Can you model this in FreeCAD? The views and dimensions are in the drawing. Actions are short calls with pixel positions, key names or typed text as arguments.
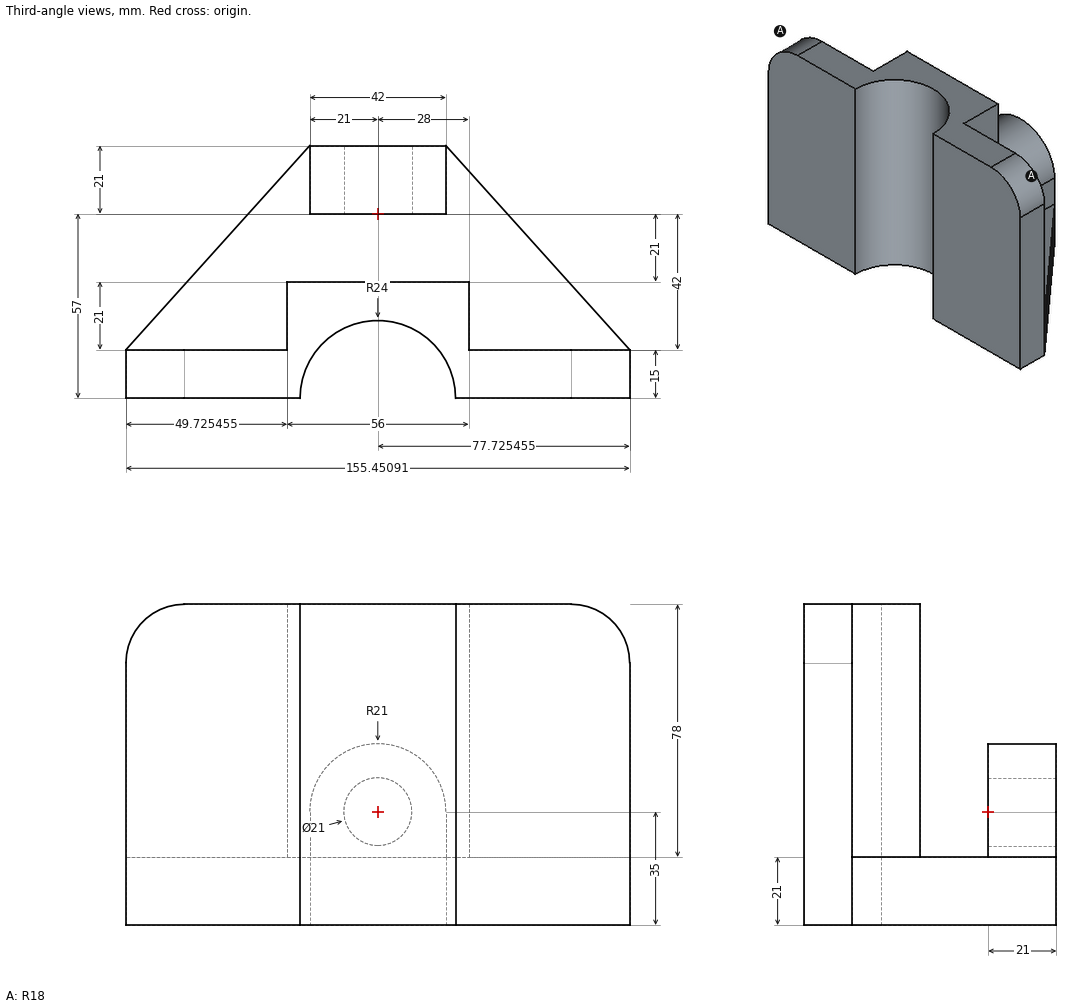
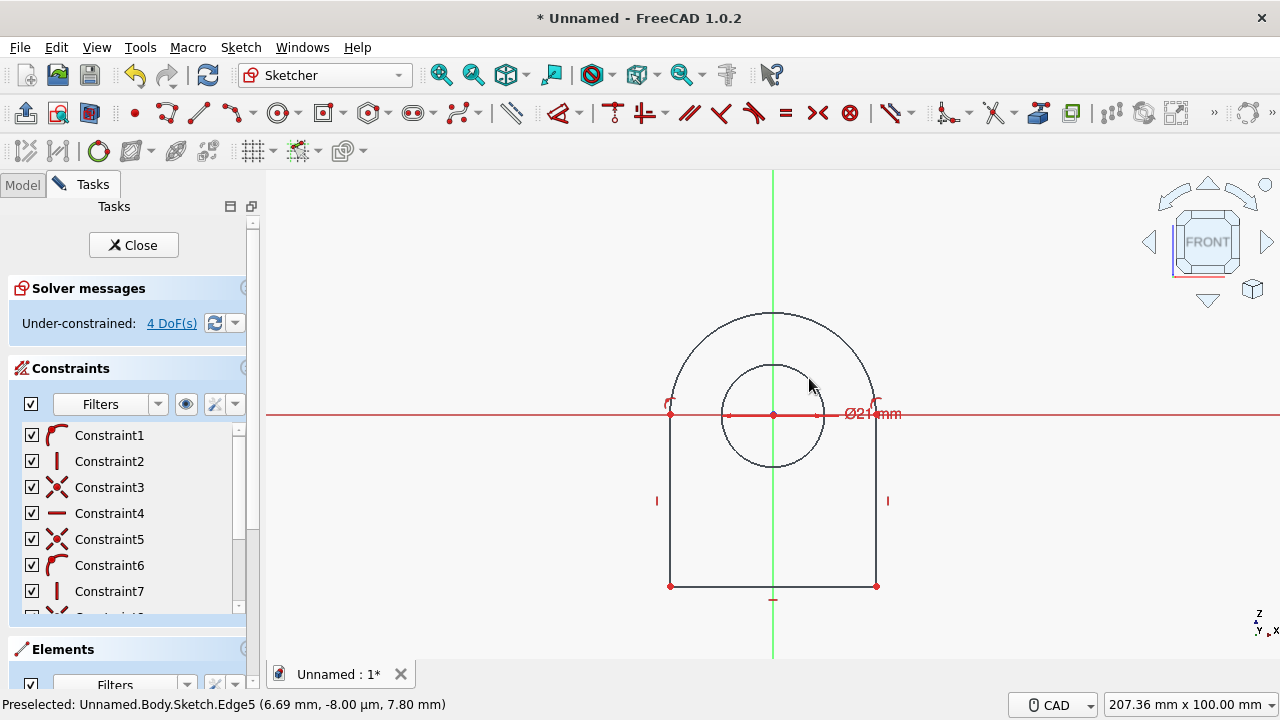
click(876, 466)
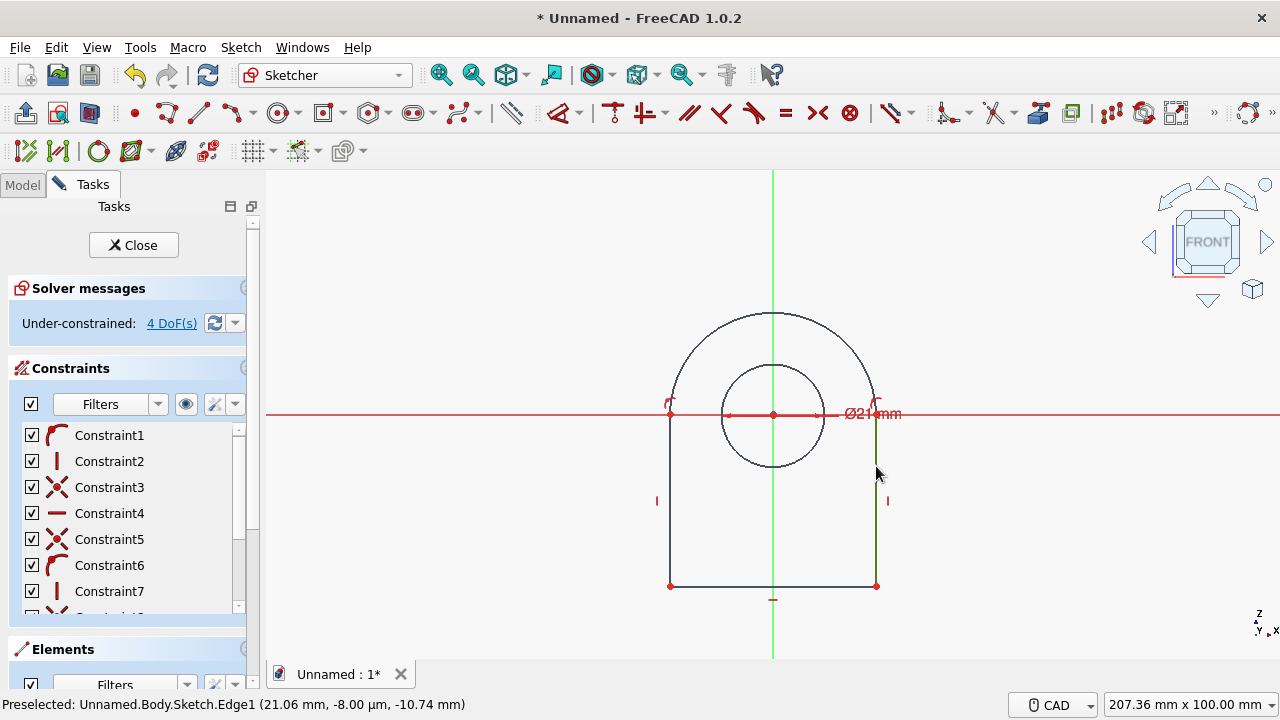
click(833, 332)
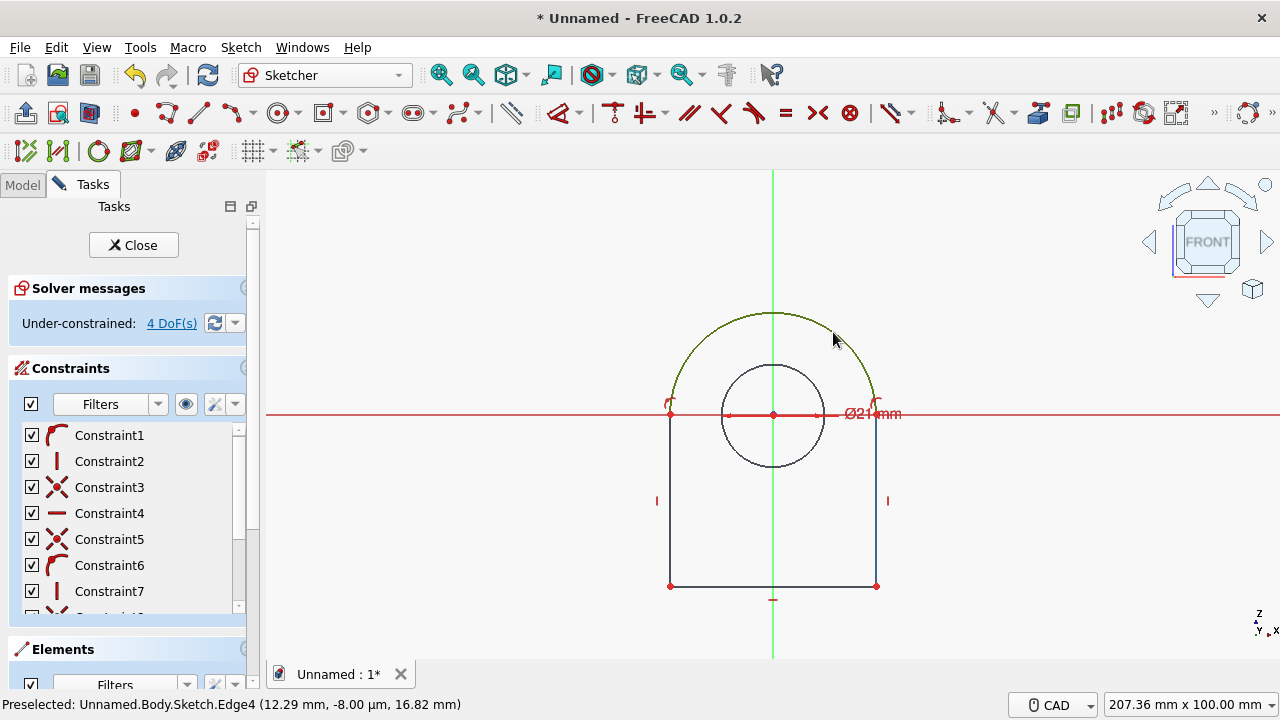
click(754, 114)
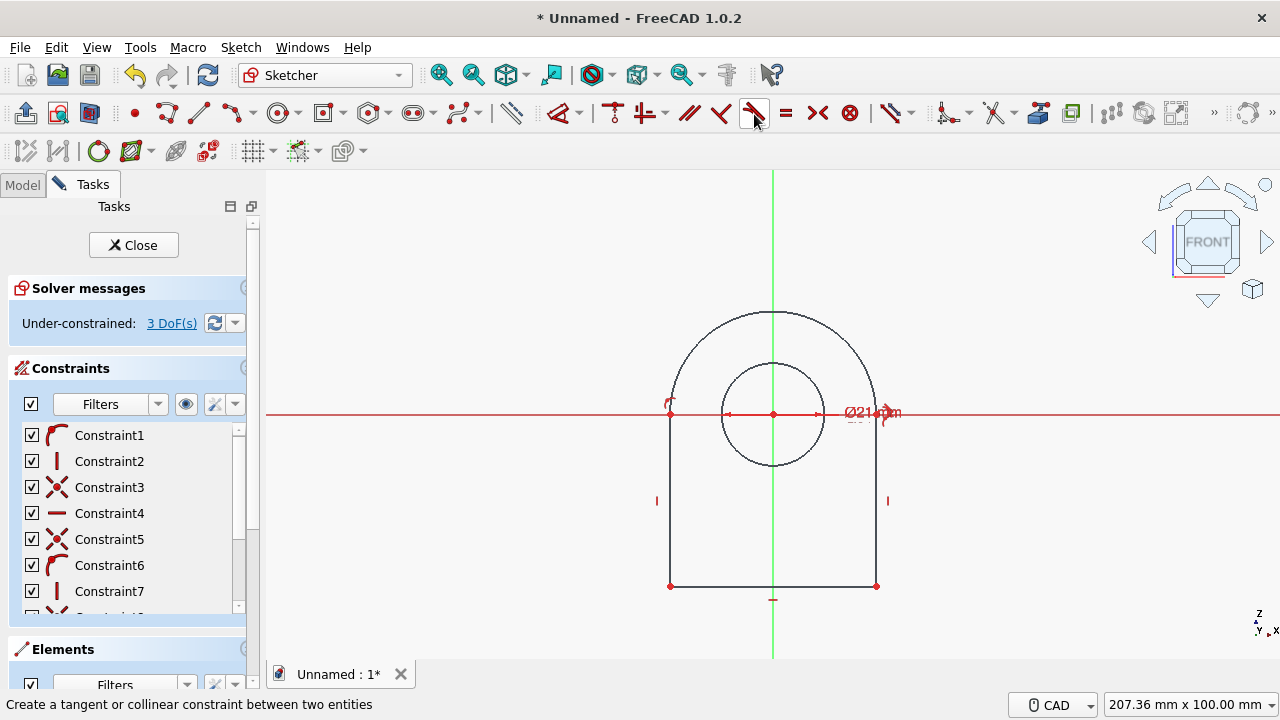
click(773, 414)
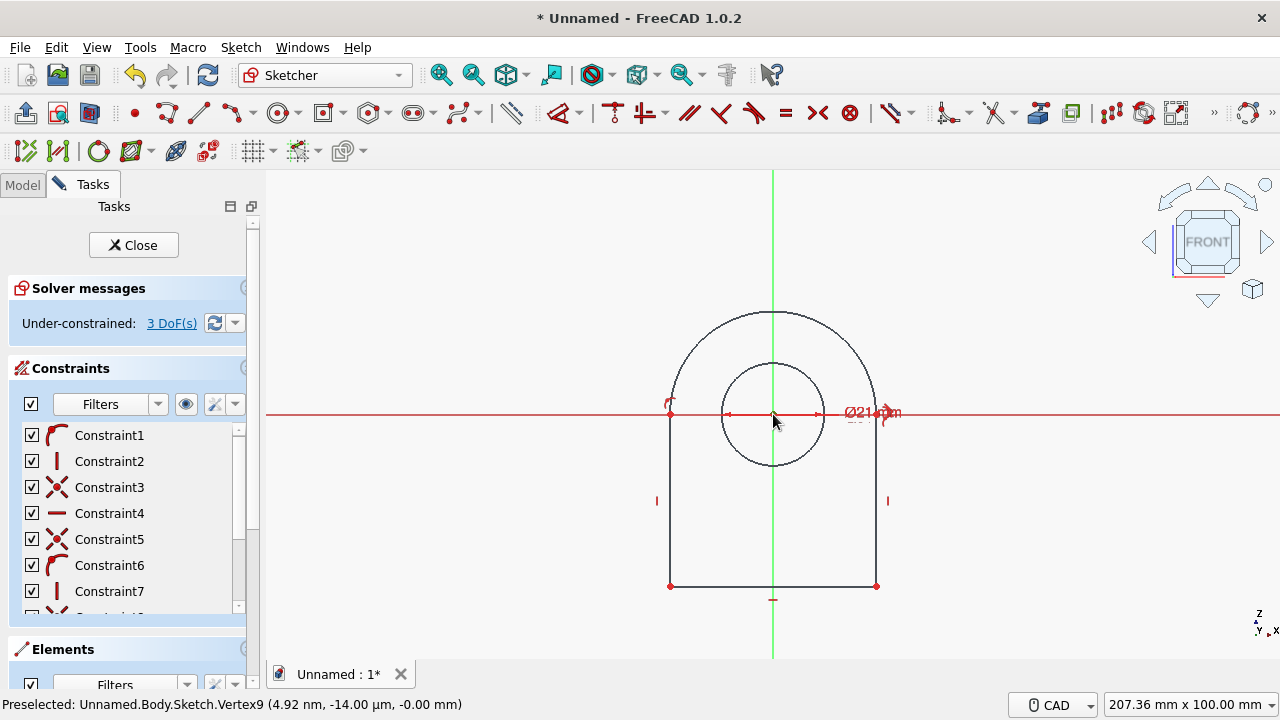
click(773, 538)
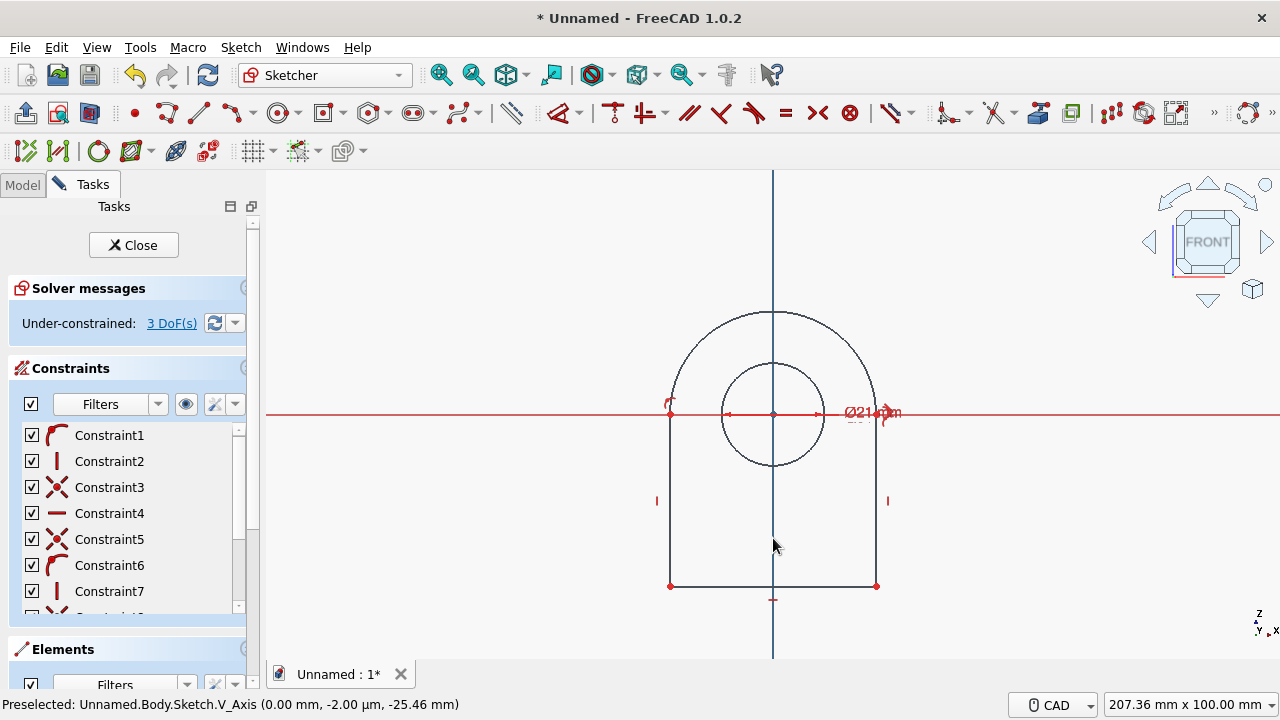
click(614, 114)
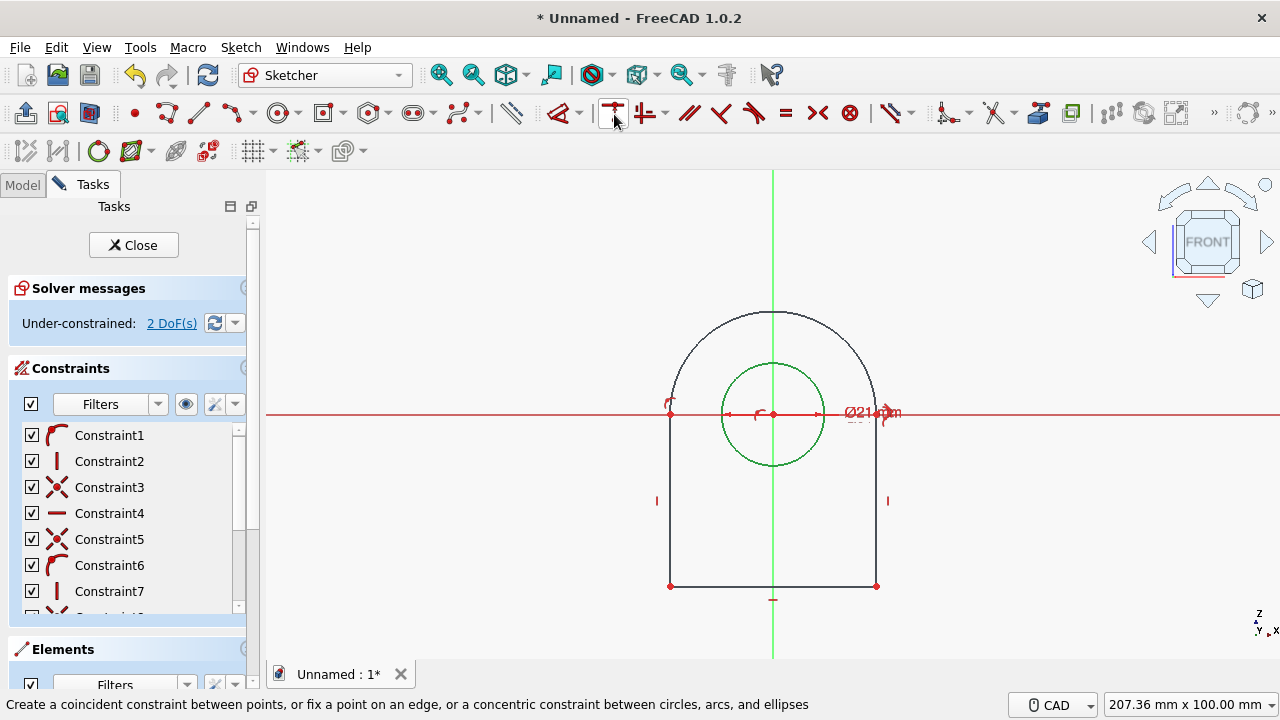
click(834, 331)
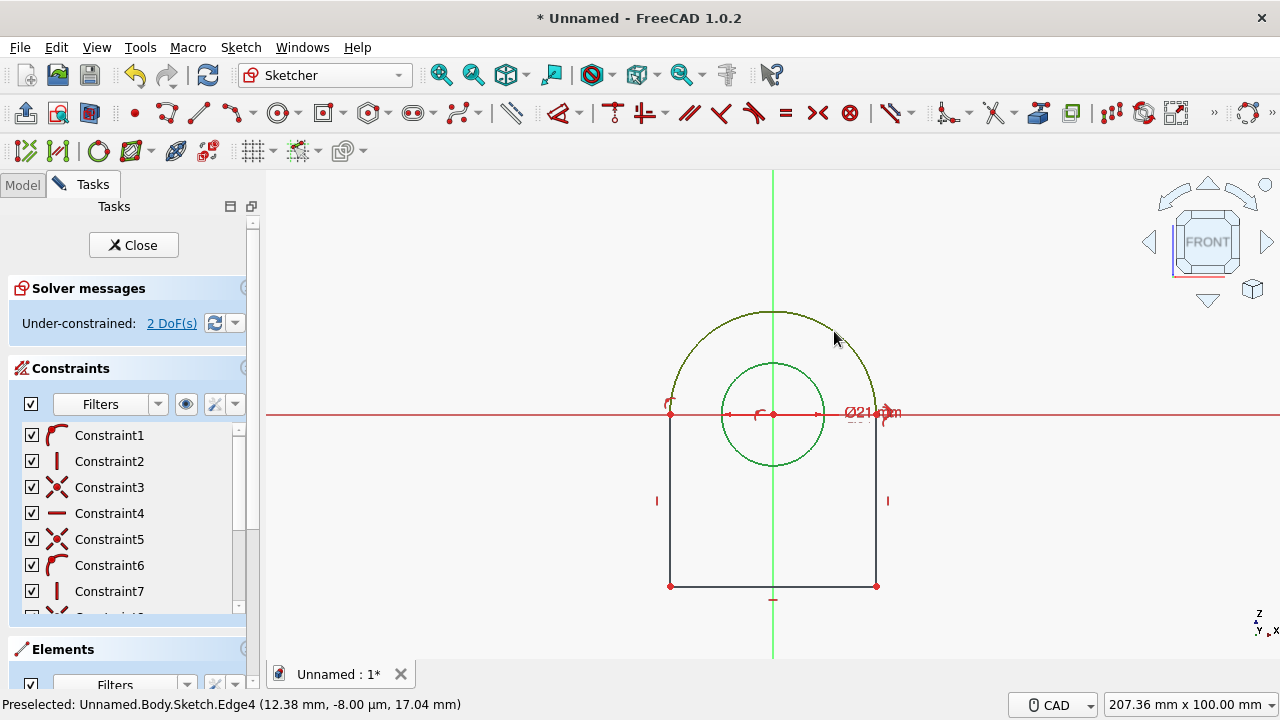
click(582, 114)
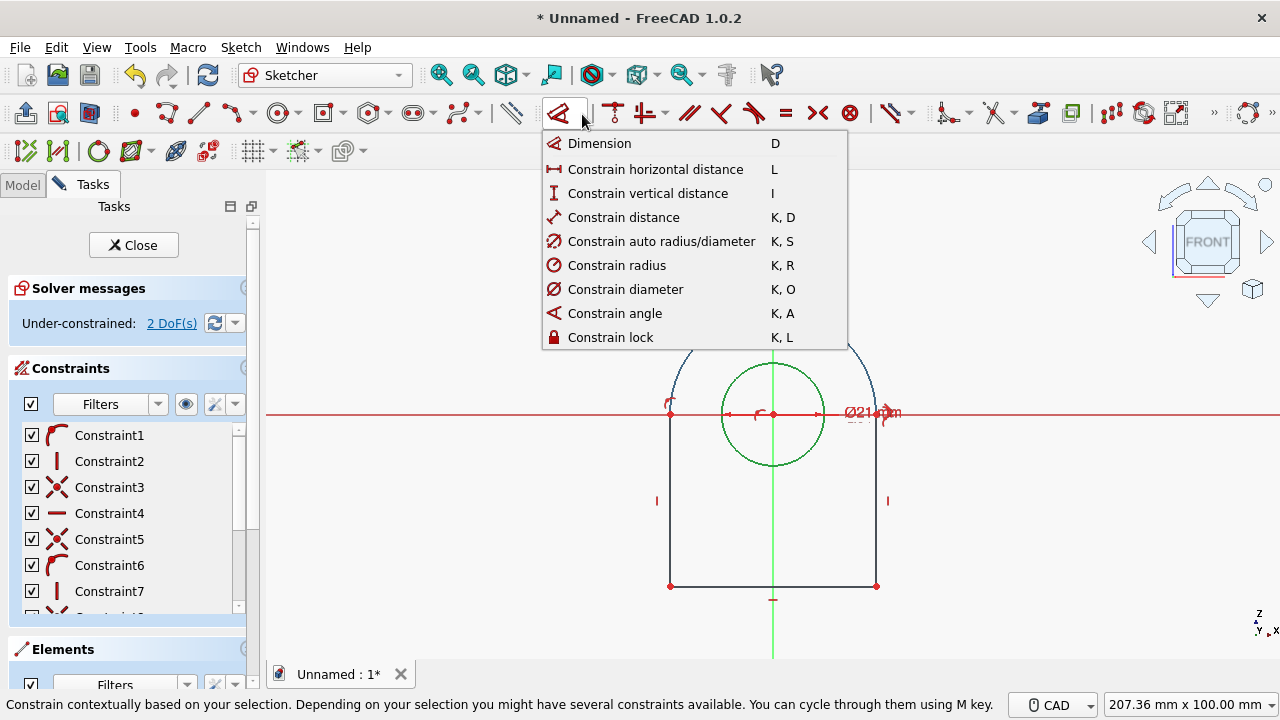
click(695, 265)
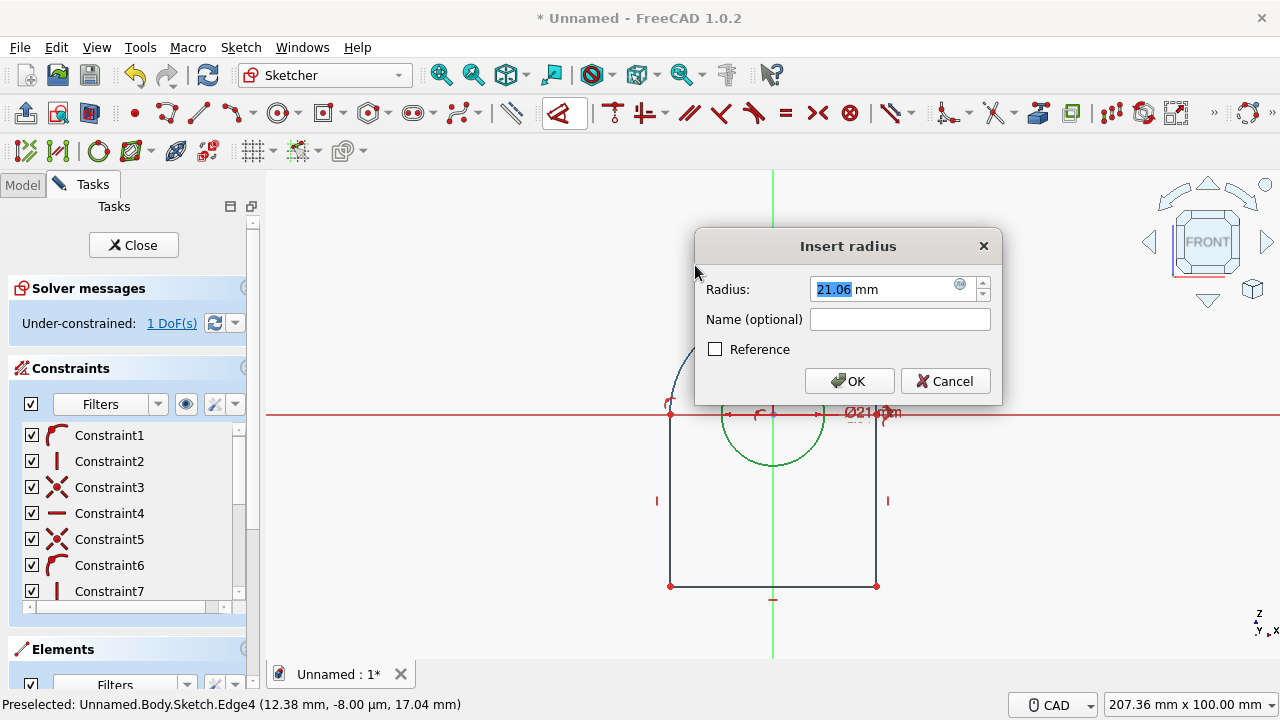
text(21)
key(Return)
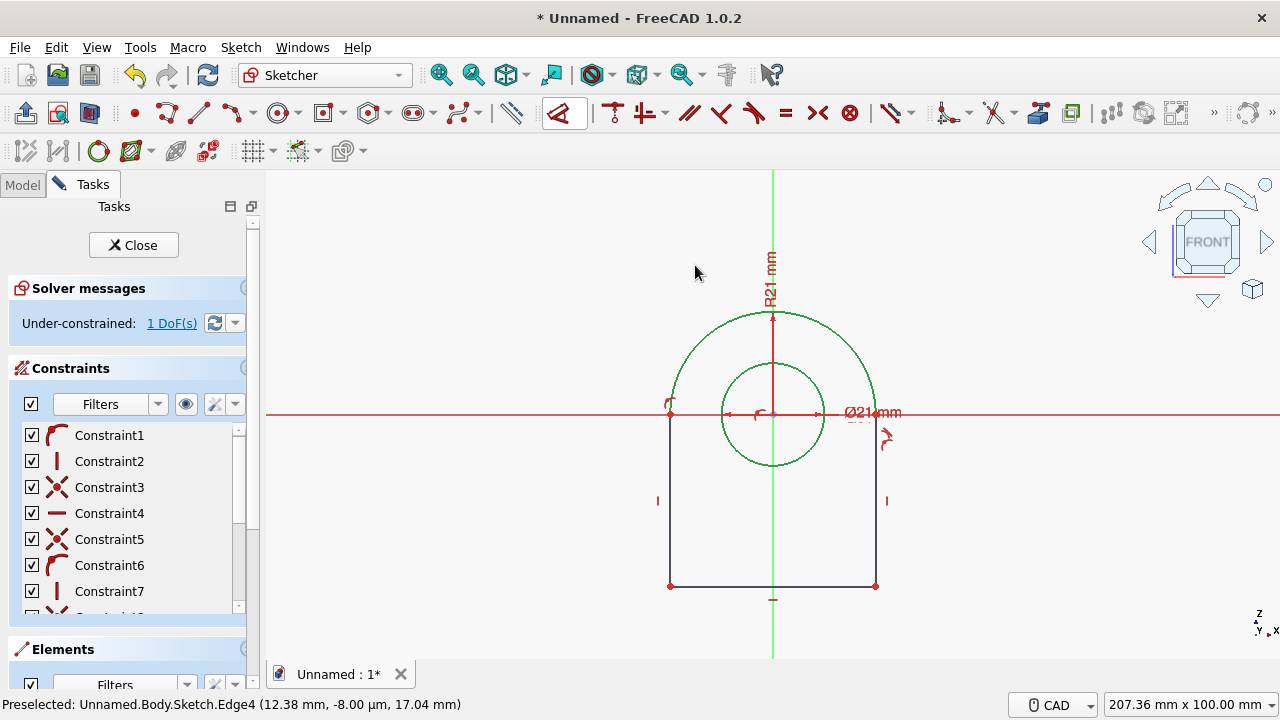
click(876, 466)